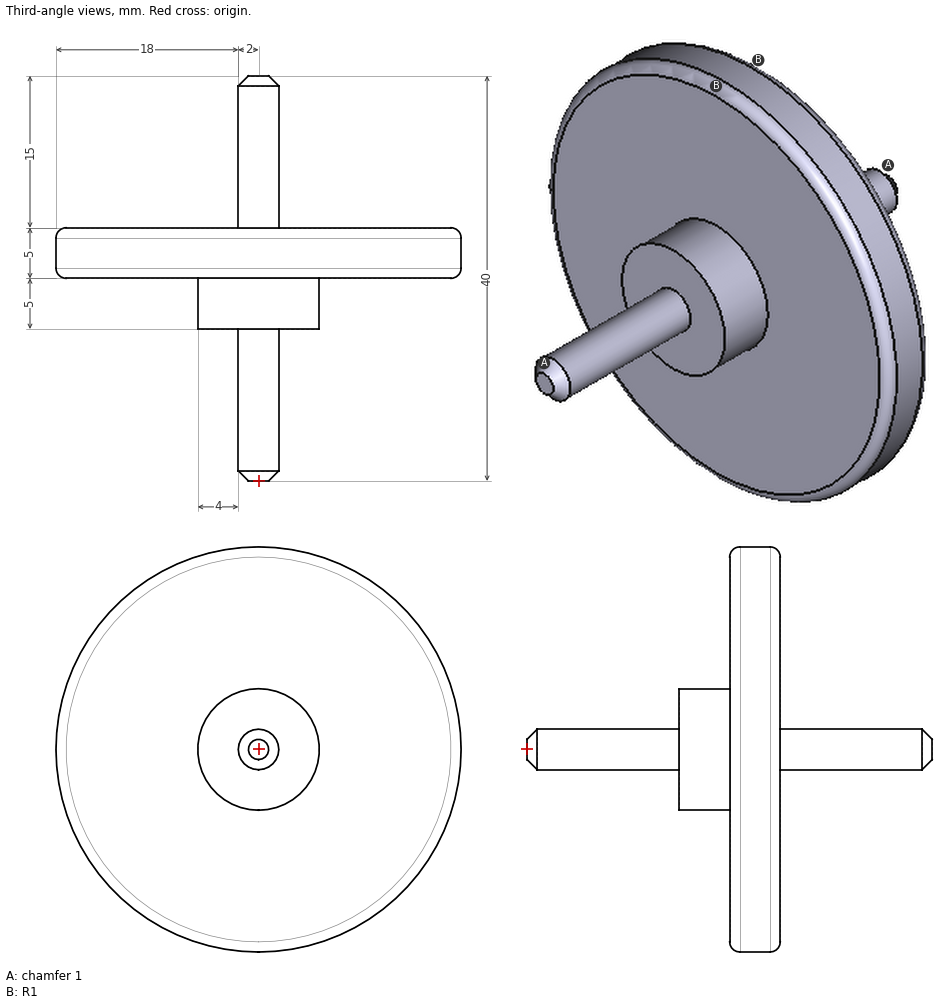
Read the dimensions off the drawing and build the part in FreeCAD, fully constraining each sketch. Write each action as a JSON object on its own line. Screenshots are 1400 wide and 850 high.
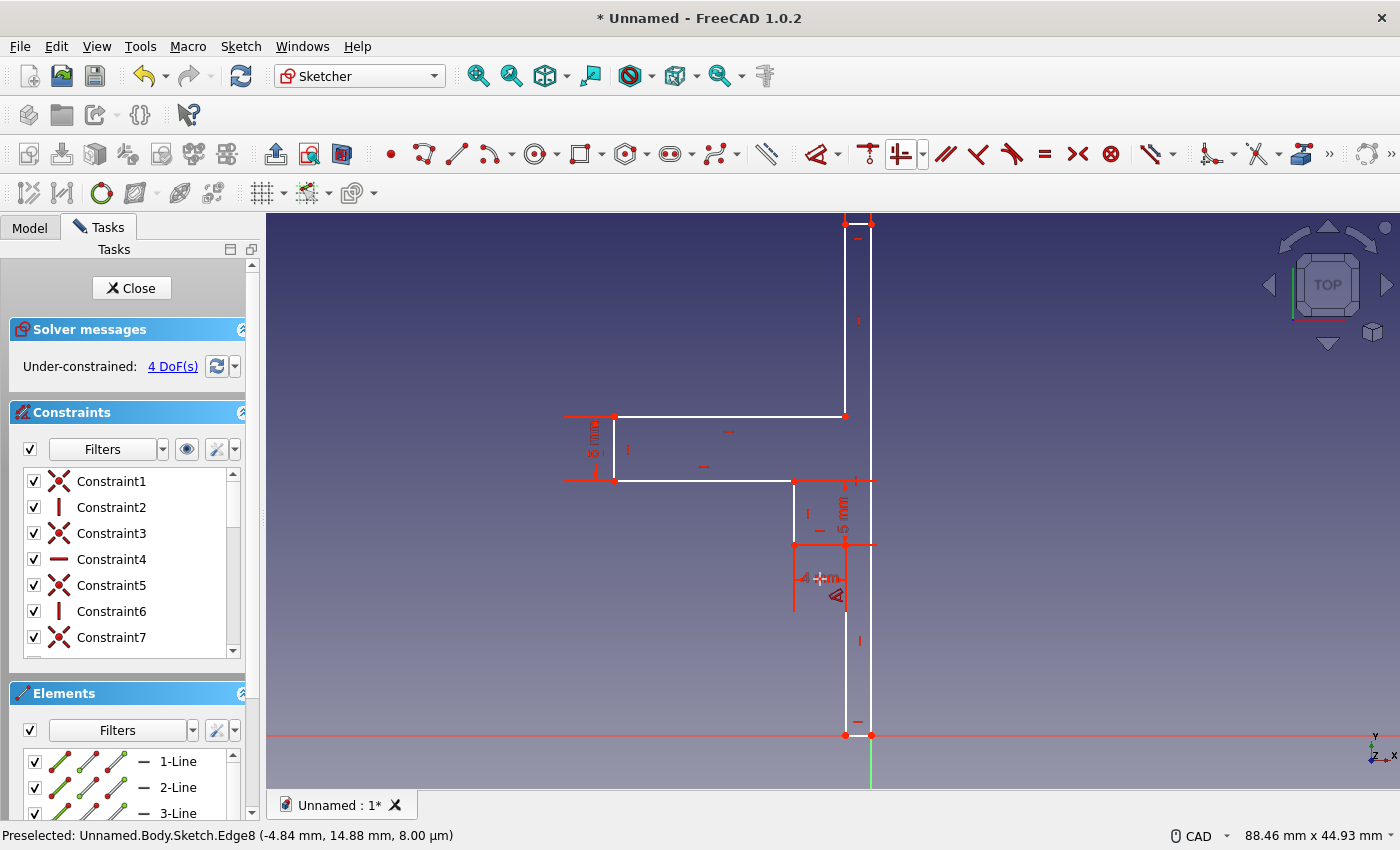
{"action": "scroll", "coordinate": [856, 736], "scroll_direction": "up", "scroll_amount": 3}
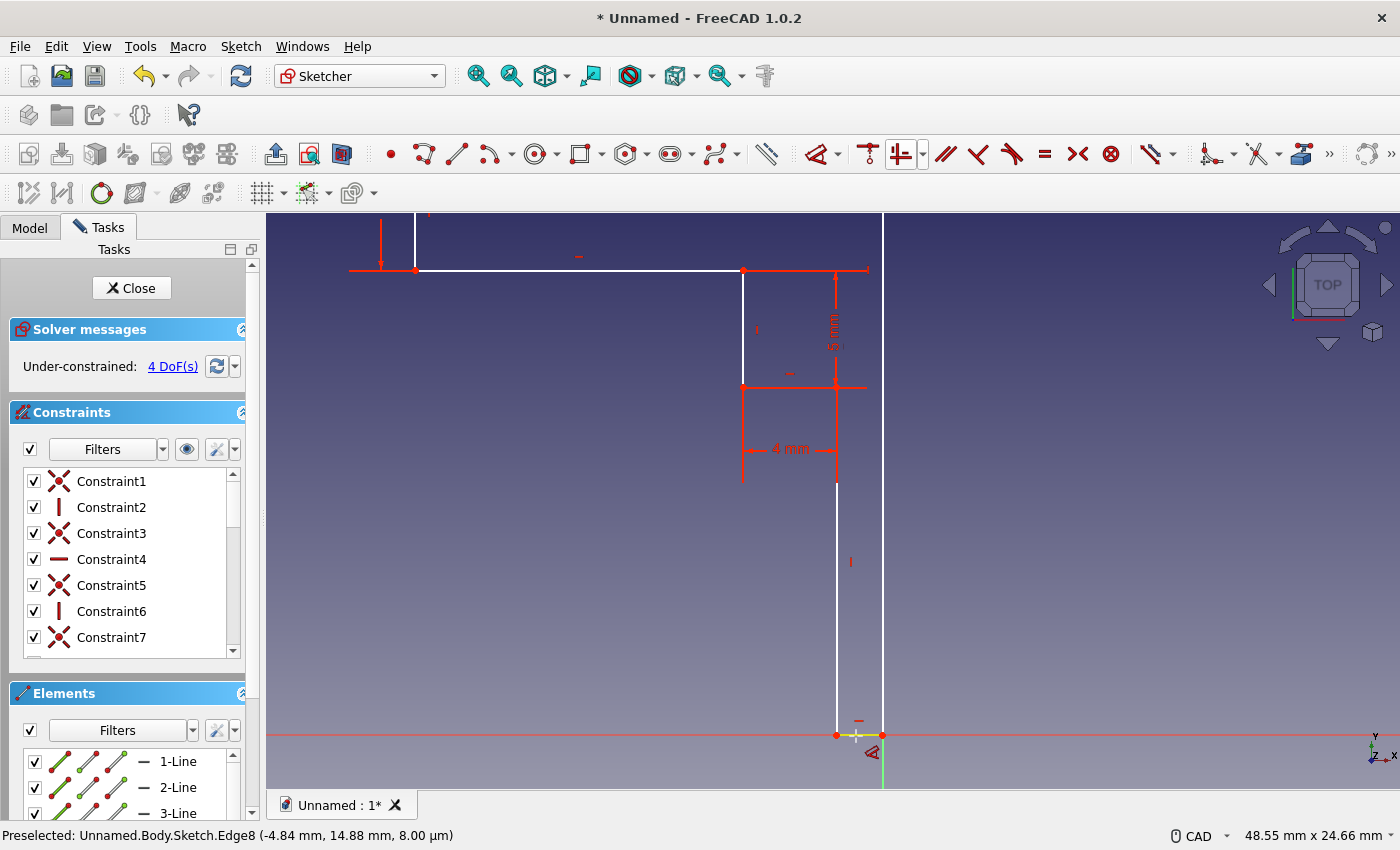
{"action": "left_click", "coordinate": [855, 735]}
{"action": "left_click", "coordinate": [860, 701]}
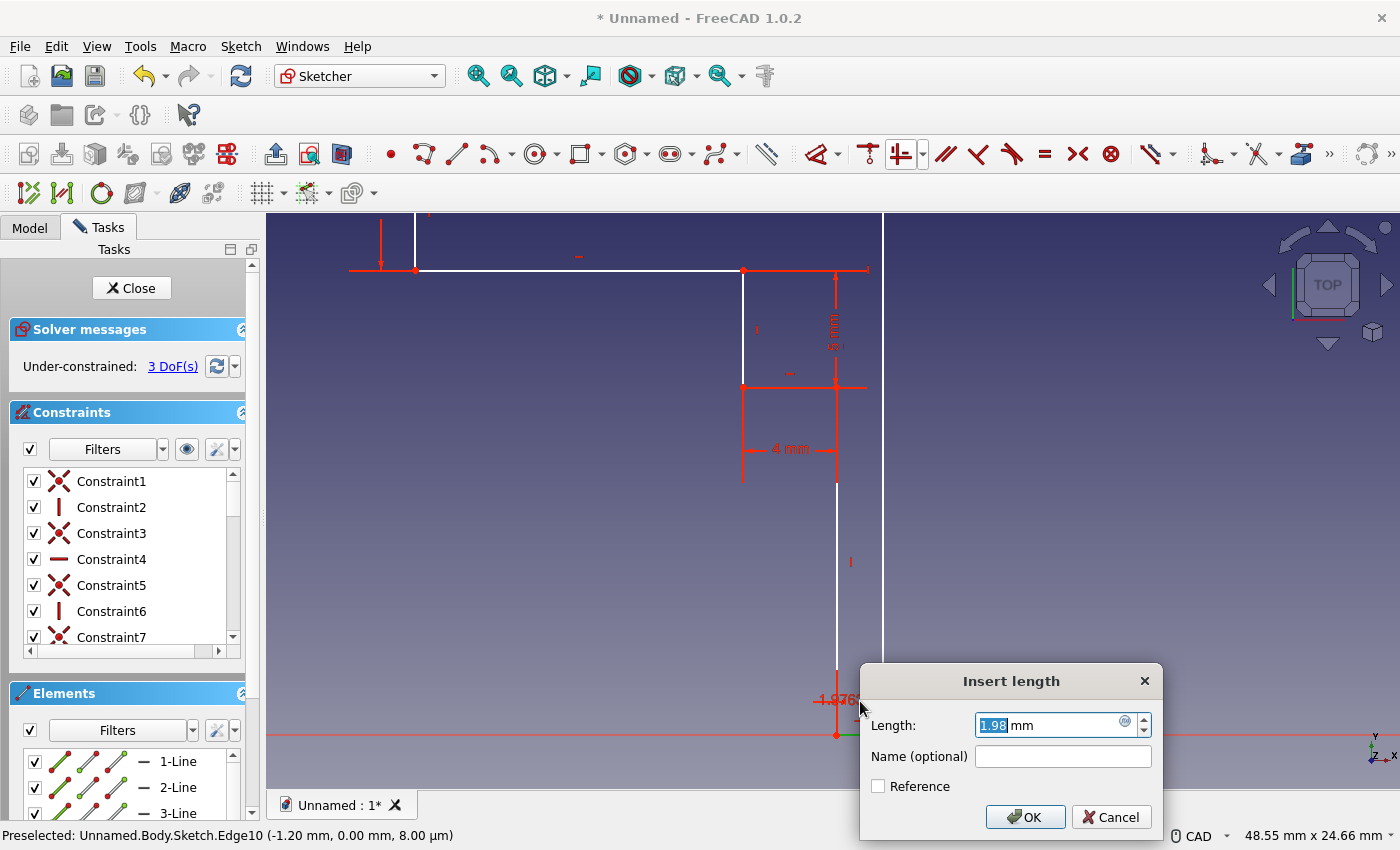
{"action": "type", "text": "2"}
{"action": "key", "text": "Return"}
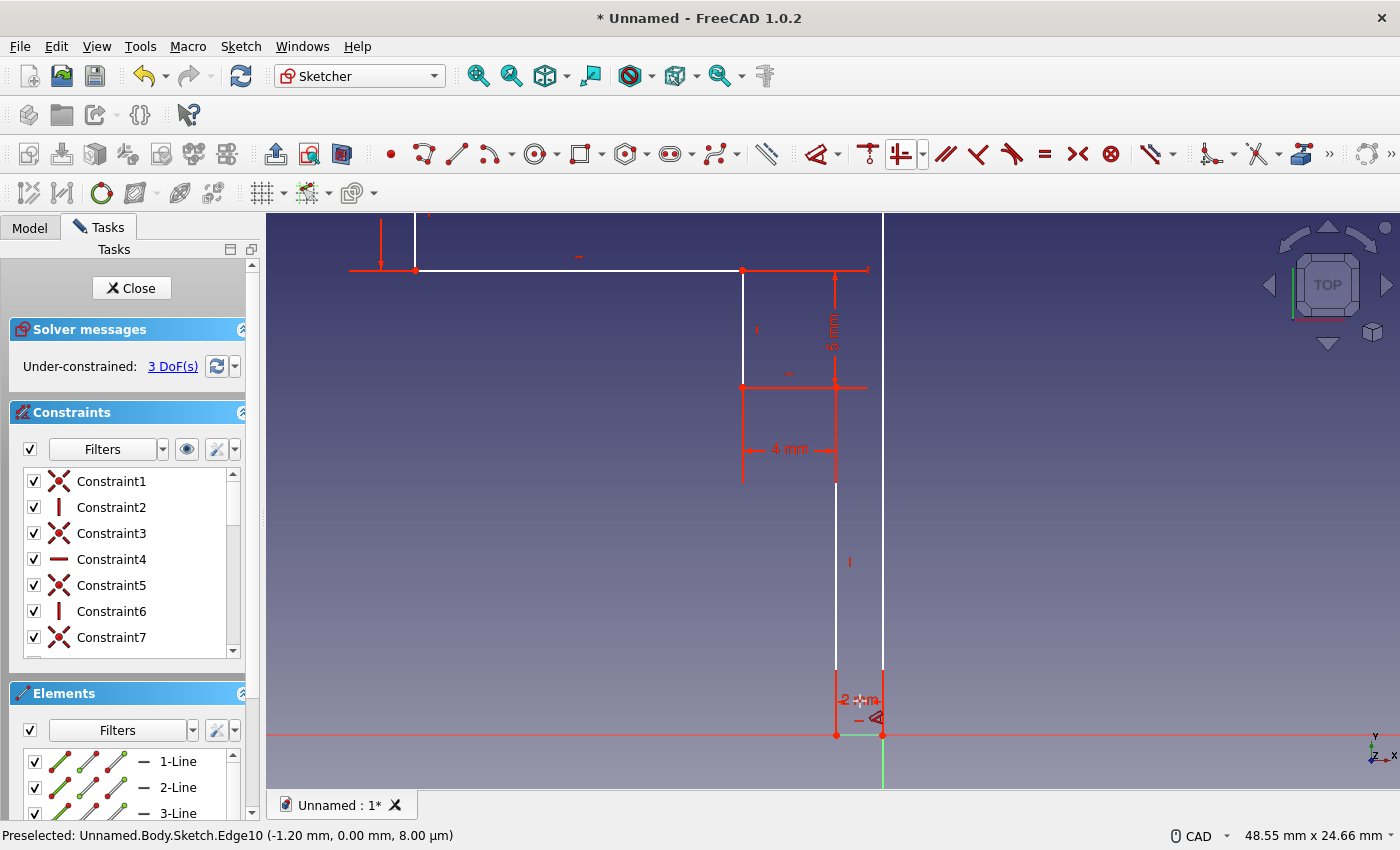
{"action": "left_click", "coordinate": [883, 455]}
{"action": "left_click", "coordinate": [917, 488]}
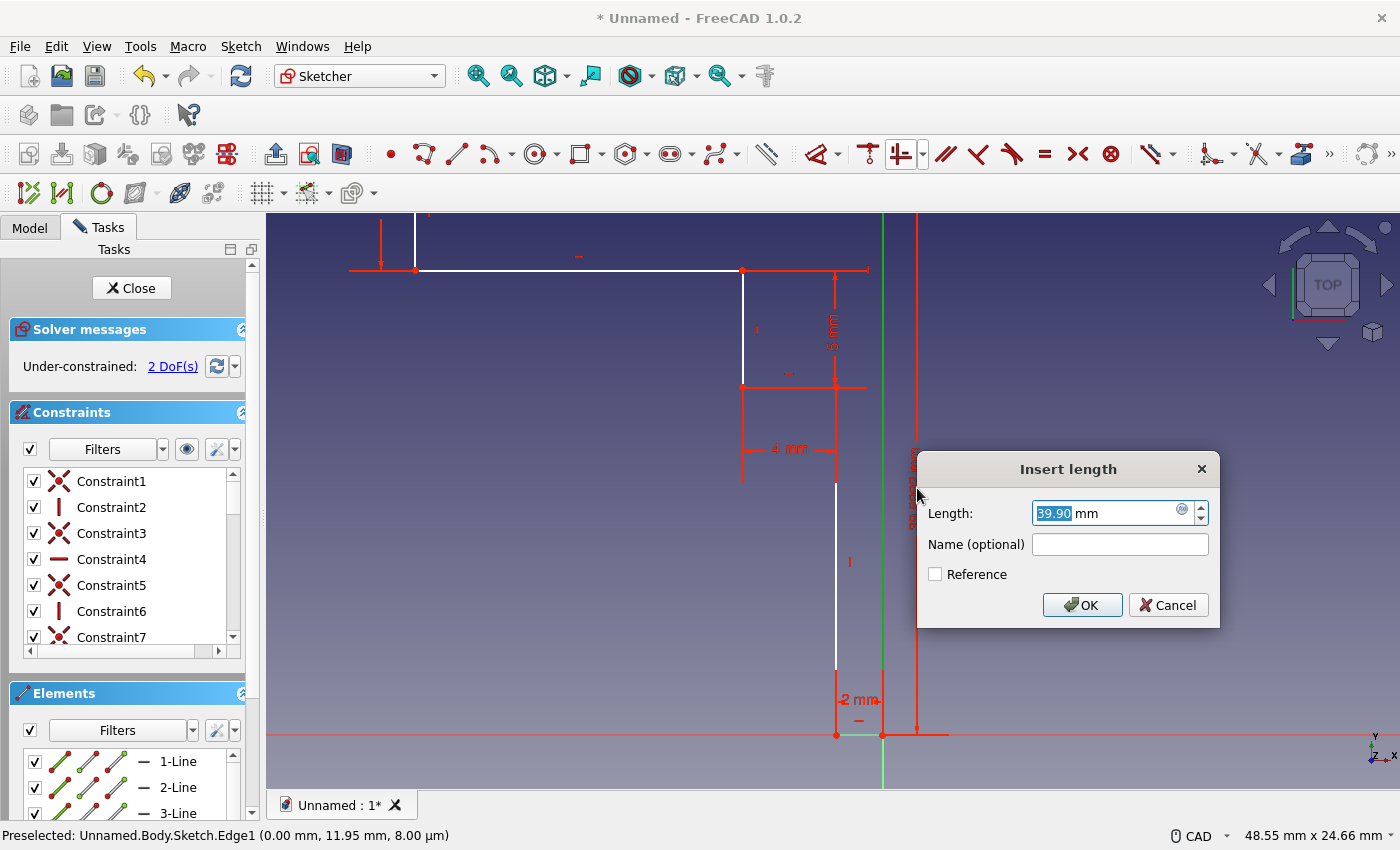
{"action": "type", "text": "40"}
{"action": "key", "text": "Return"}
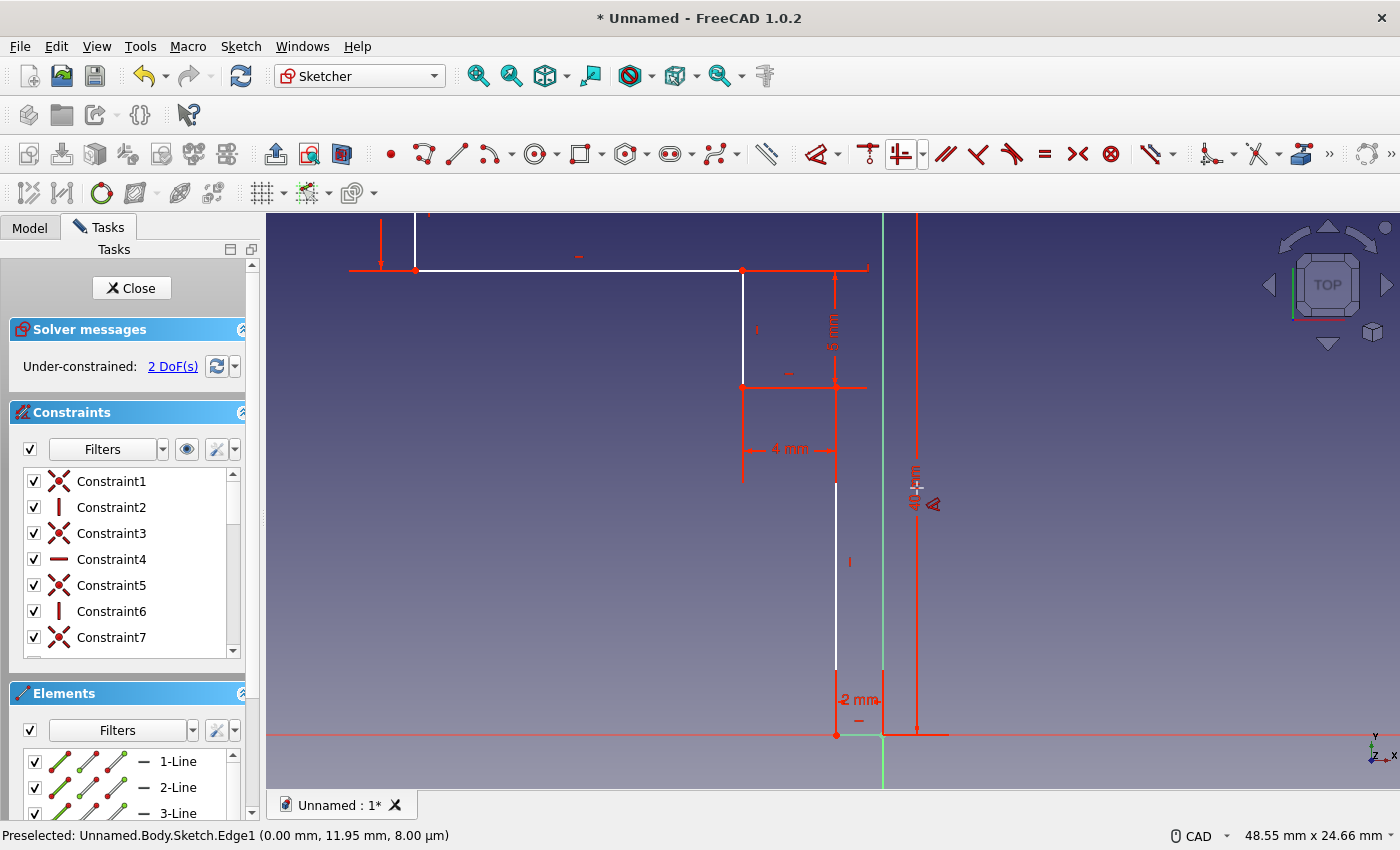
{"action": "scroll", "coordinate": [831, 637], "scroll_direction": "down", "scroll_amount": 5}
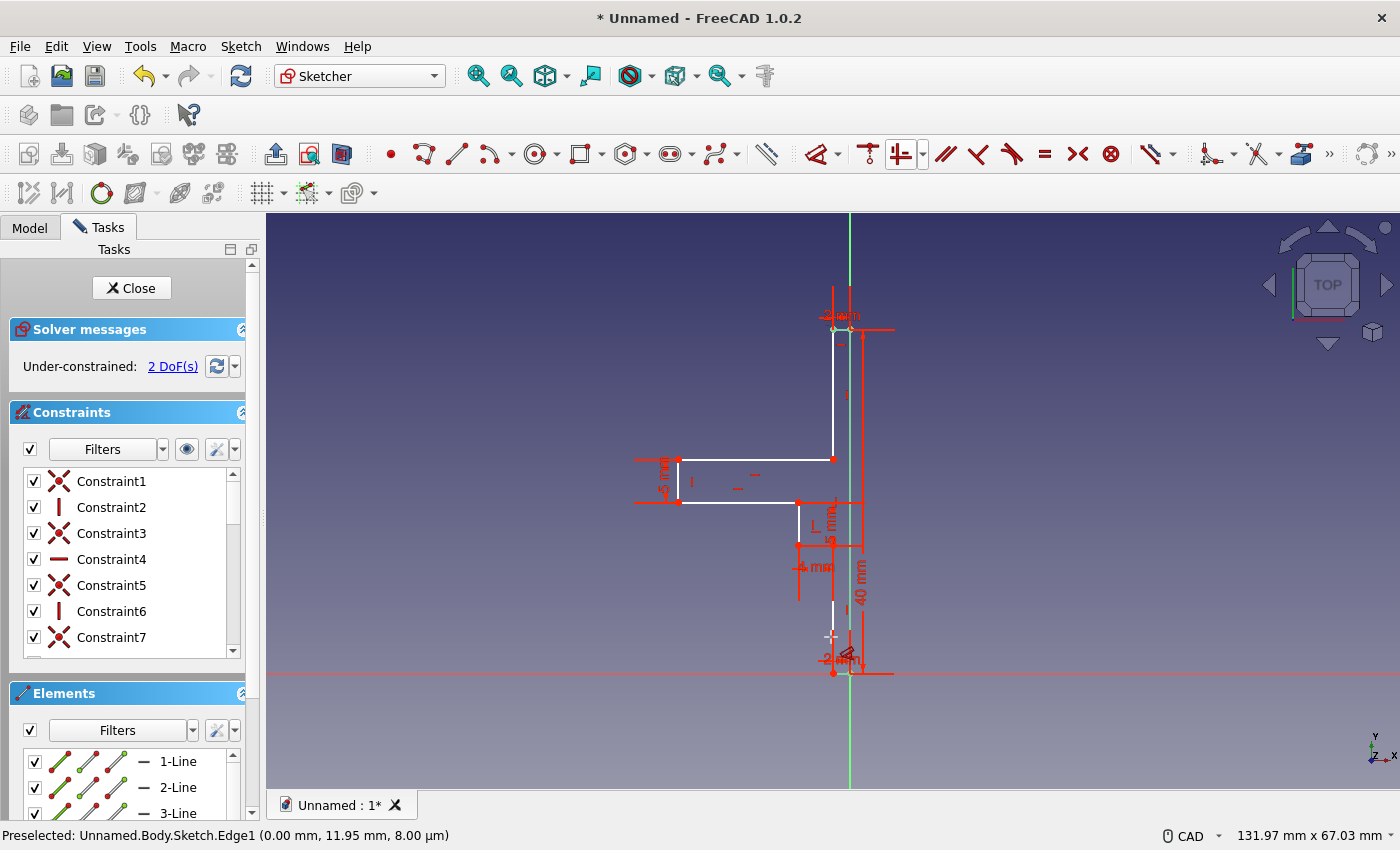
{"action": "left_click", "coordinate": [833, 369]}
{"action": "left_click", "coordinate": [867, 395]}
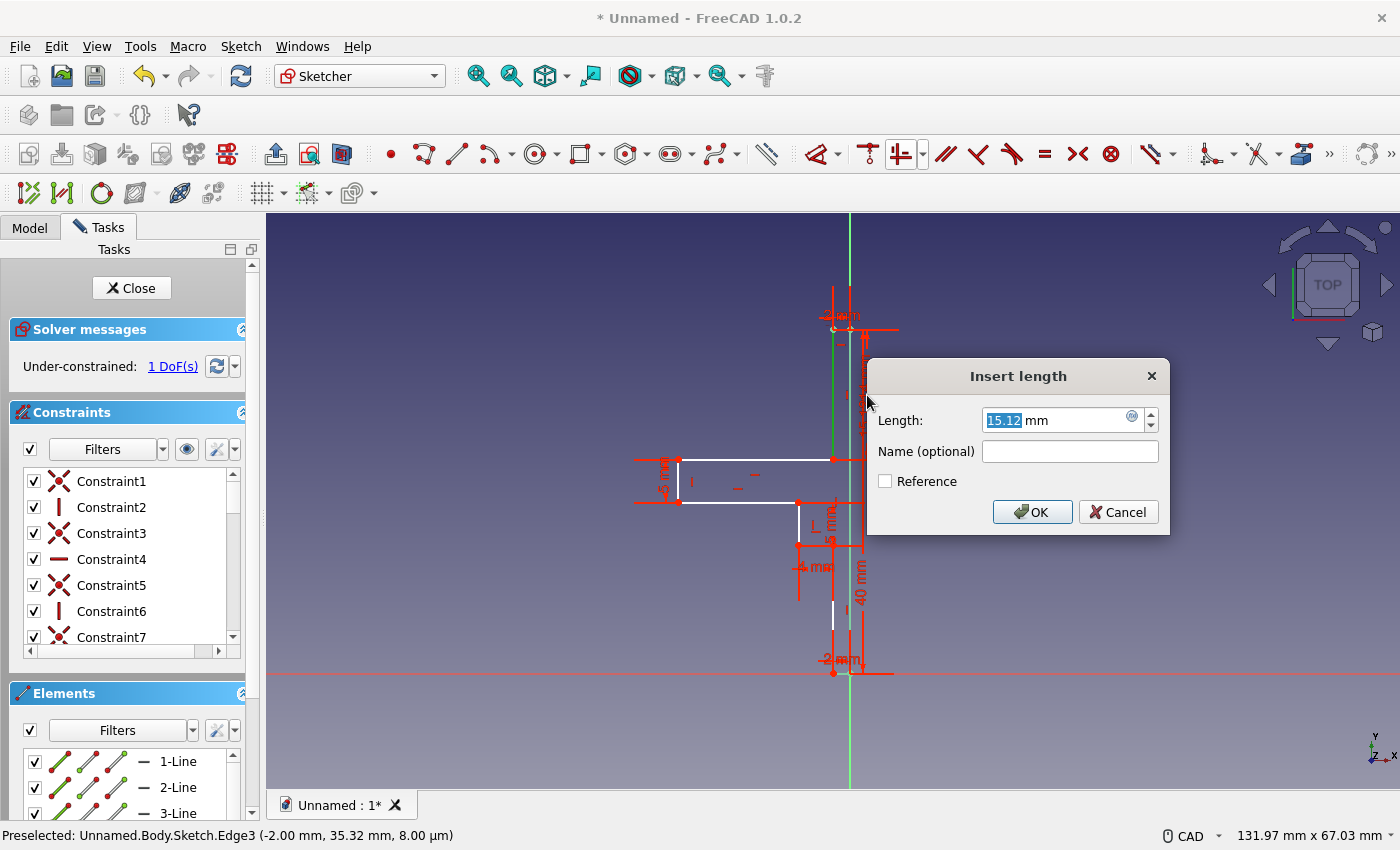
{"action": "type", "text": "15"}
{"action": "key", "text": "Return"}